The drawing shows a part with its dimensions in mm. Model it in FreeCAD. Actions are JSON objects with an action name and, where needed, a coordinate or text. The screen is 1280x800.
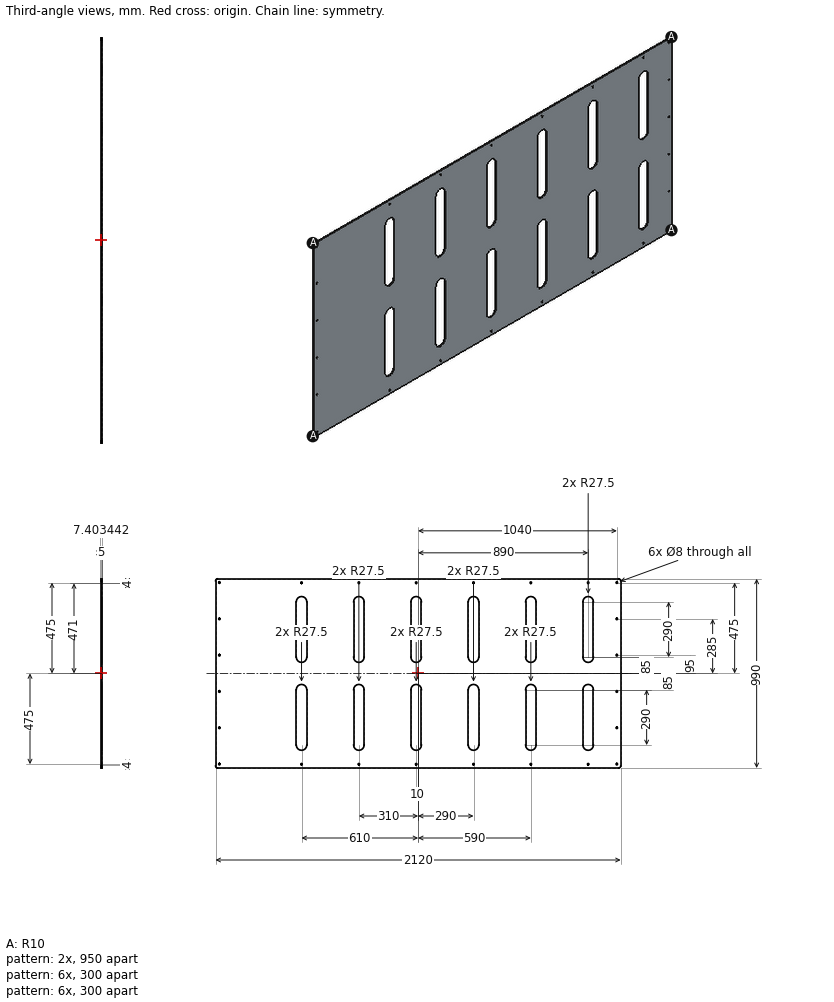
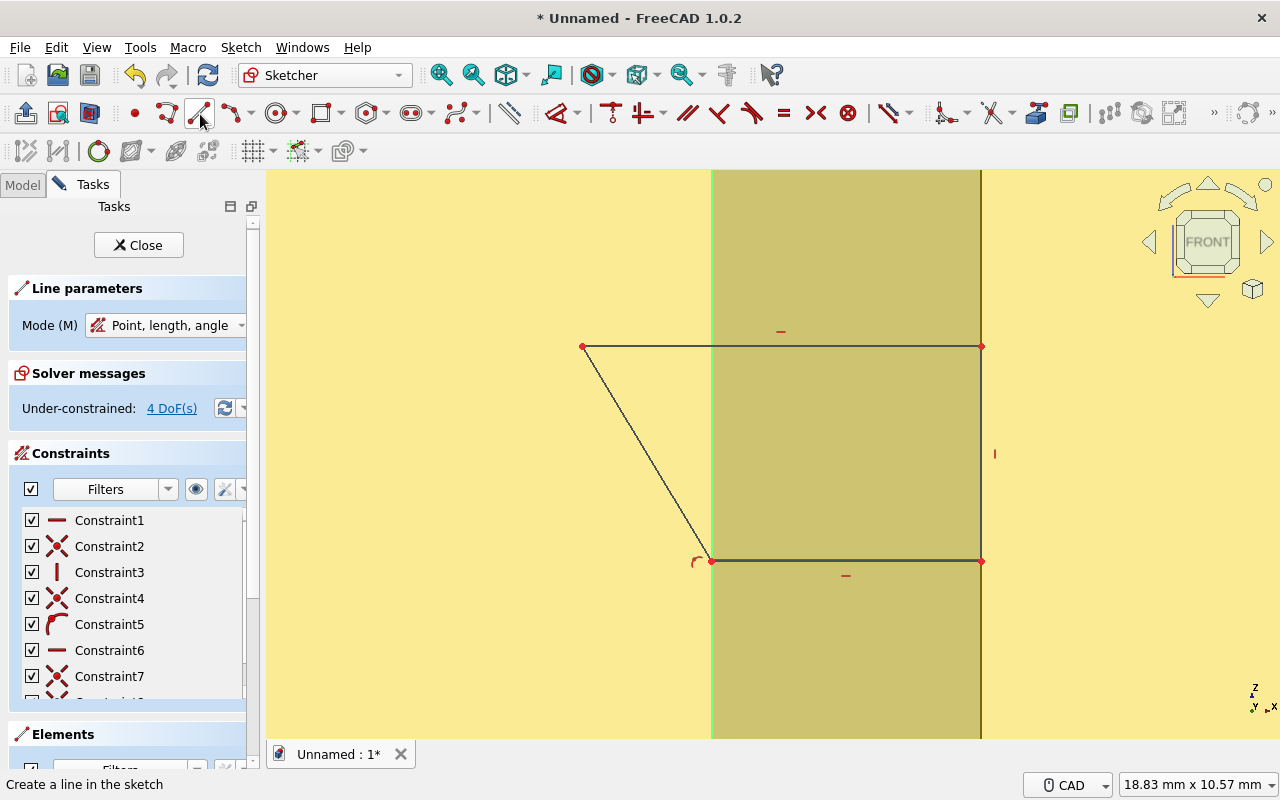
{"action": "left_click", "coordinate": [542, 345]}
{"action": "left_click", "coordinate": [423, 345]}
{"action": "key", "text": "Escape"}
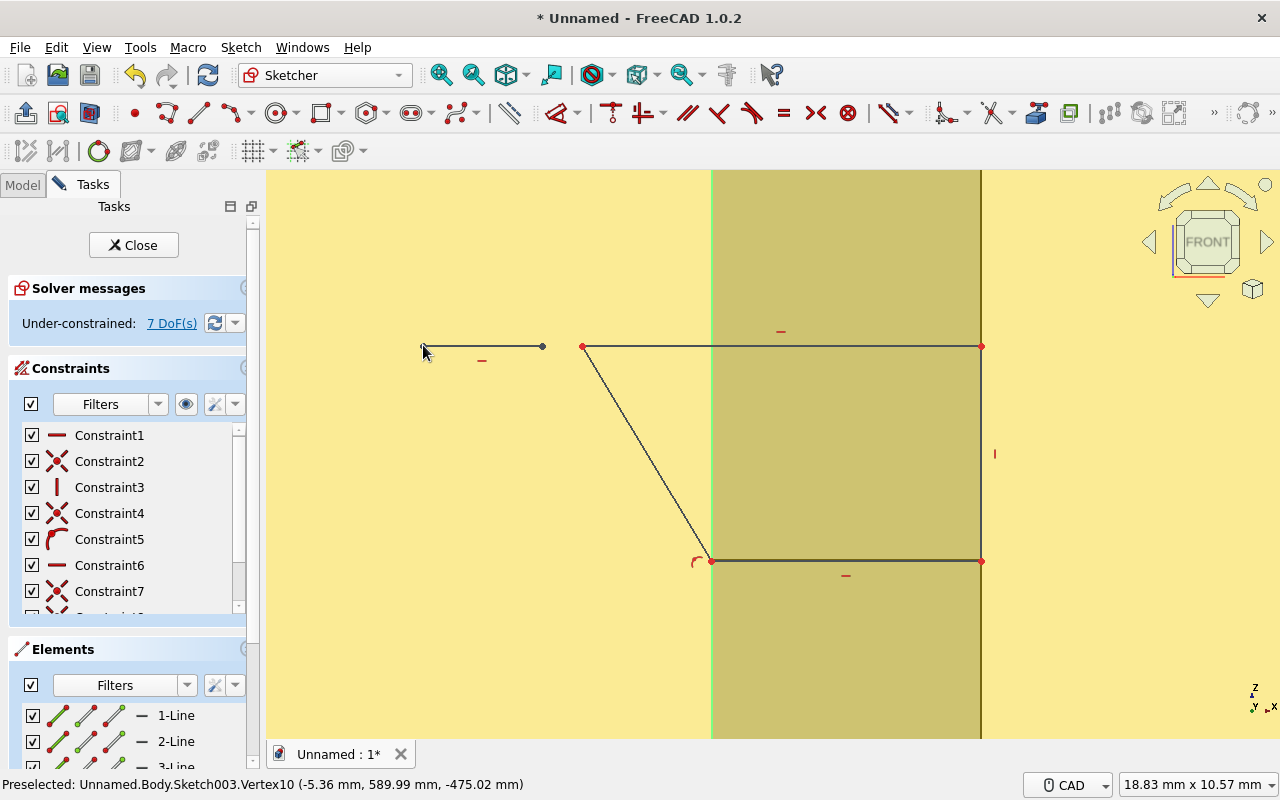
{"action": "left_click", "coordinate": [506, 346]}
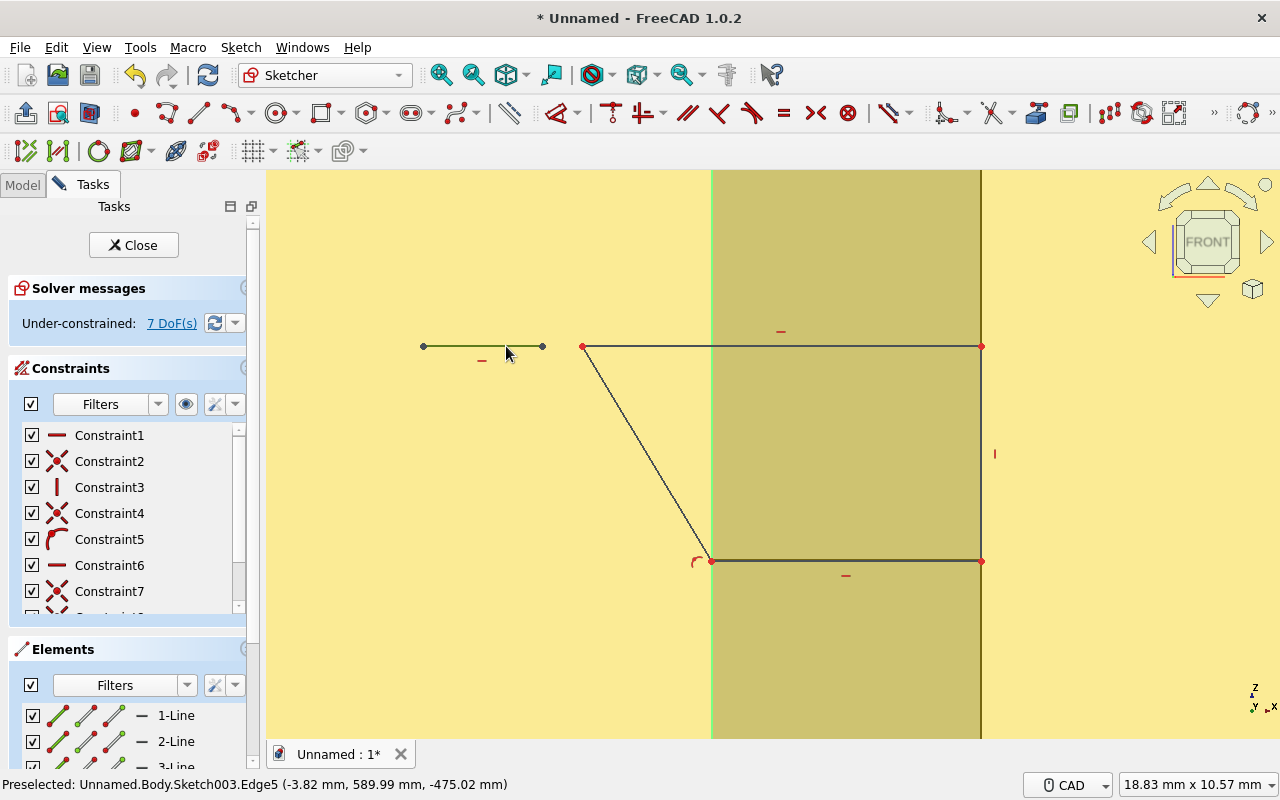
{"action": "key", "text": "g n"}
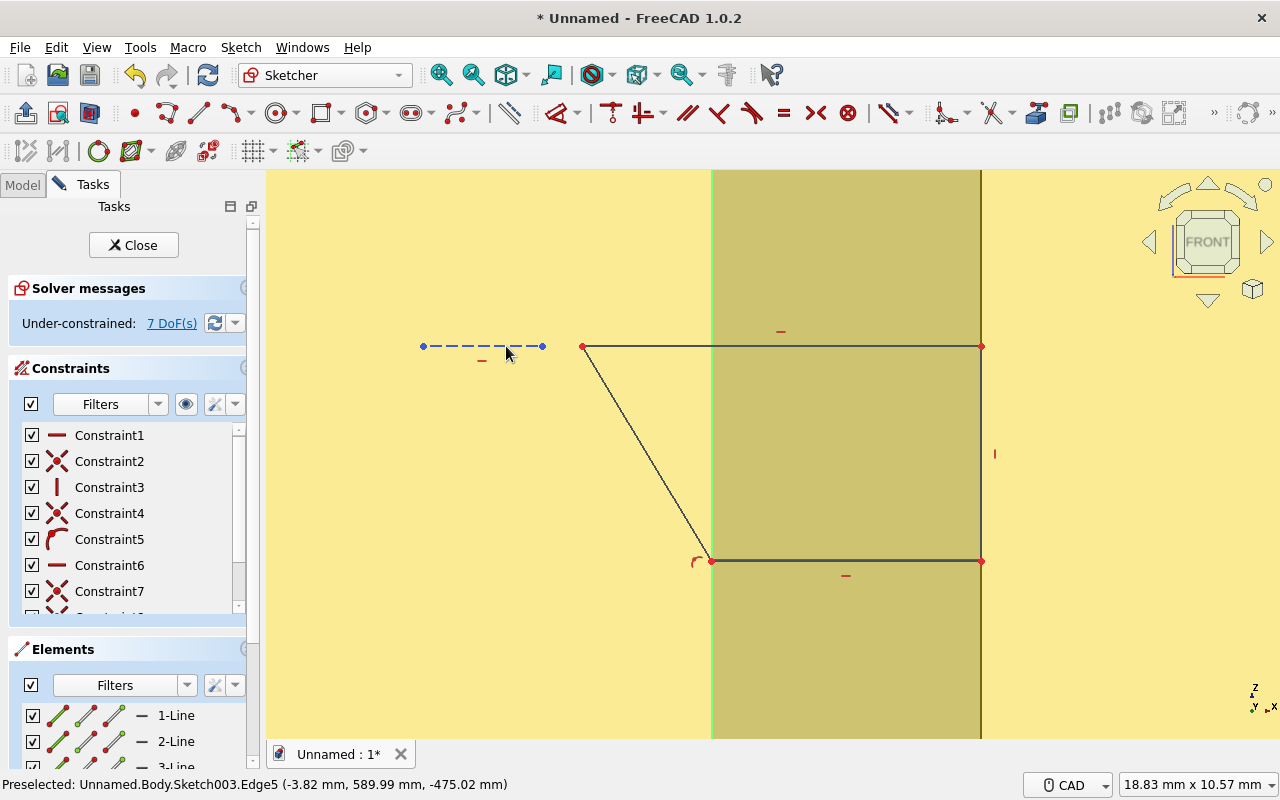
{"action": "key", "text": "d"}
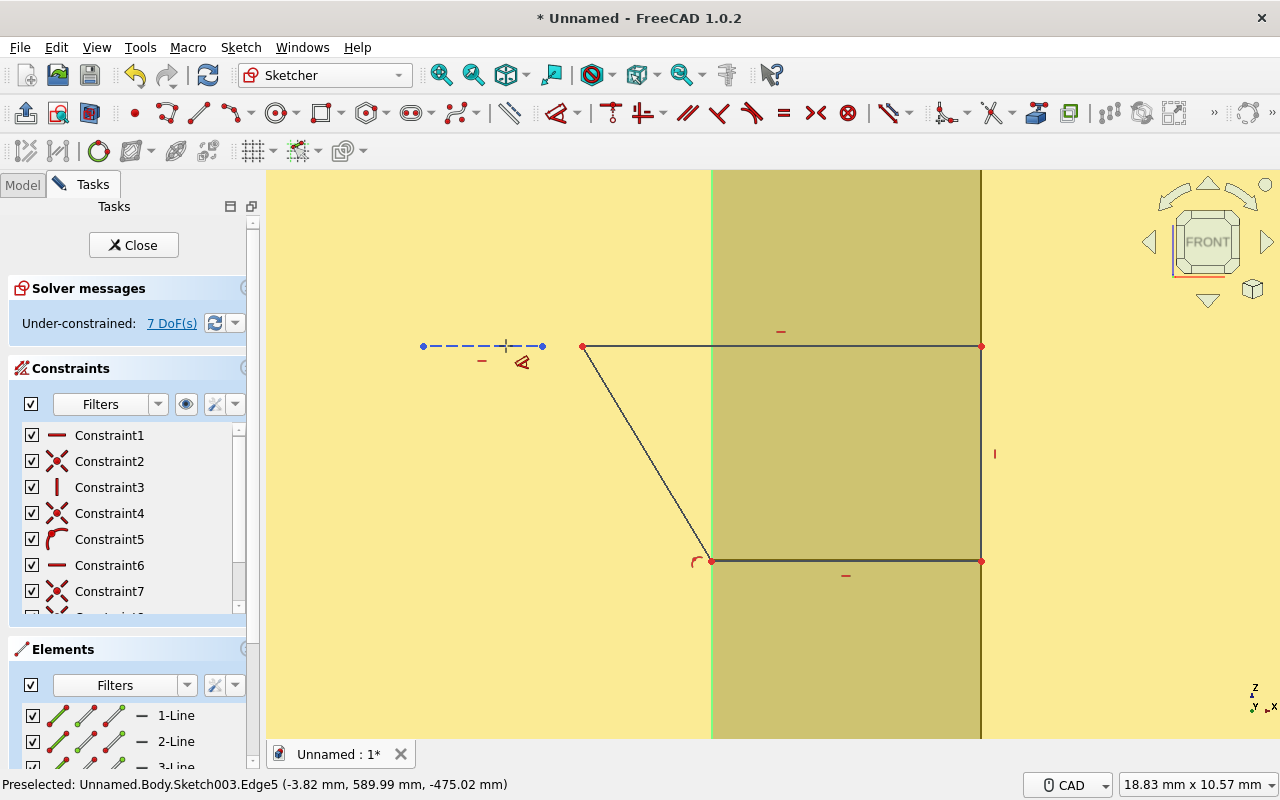
{"action": "left_click", "coordinate": [981, 411]}
{"action": "left_click", "coordinate": [1015, 454]}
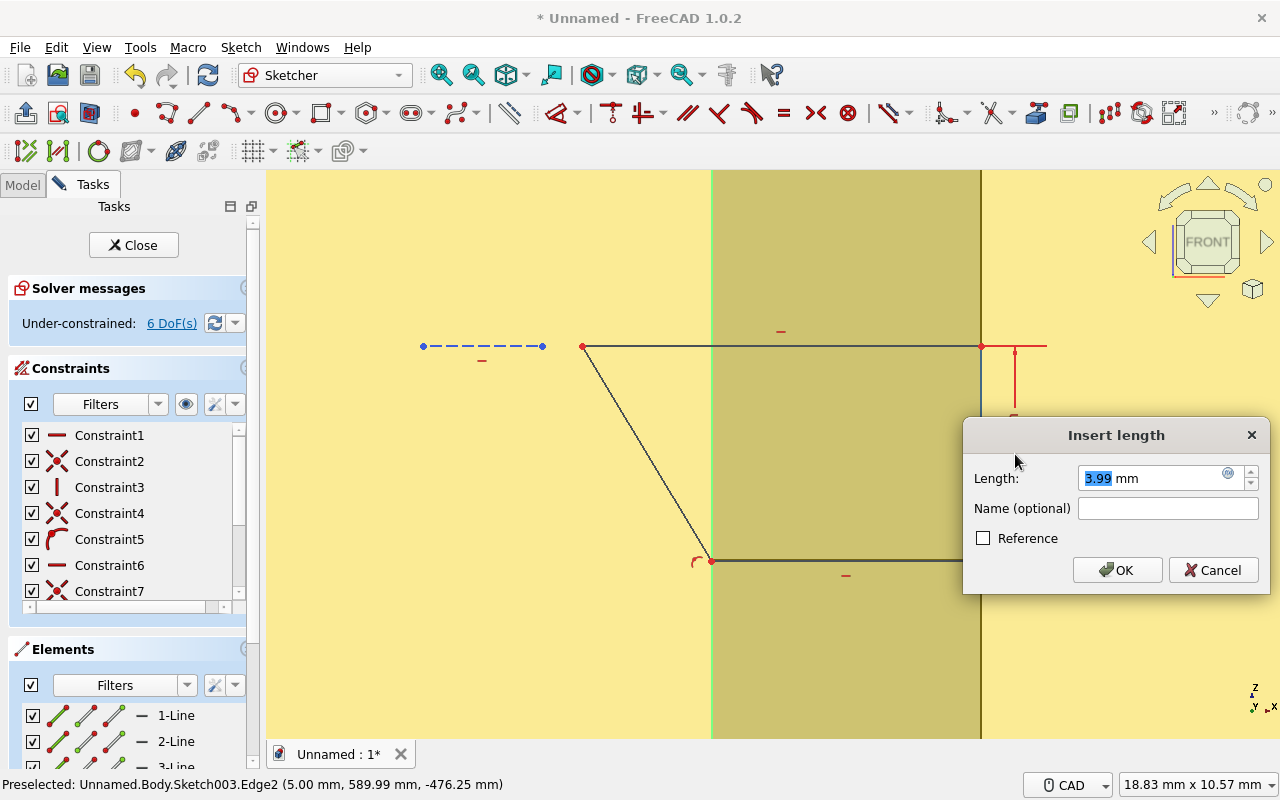
{"action": "type", "text": "4"}
{"action": "key", "text": "Return"}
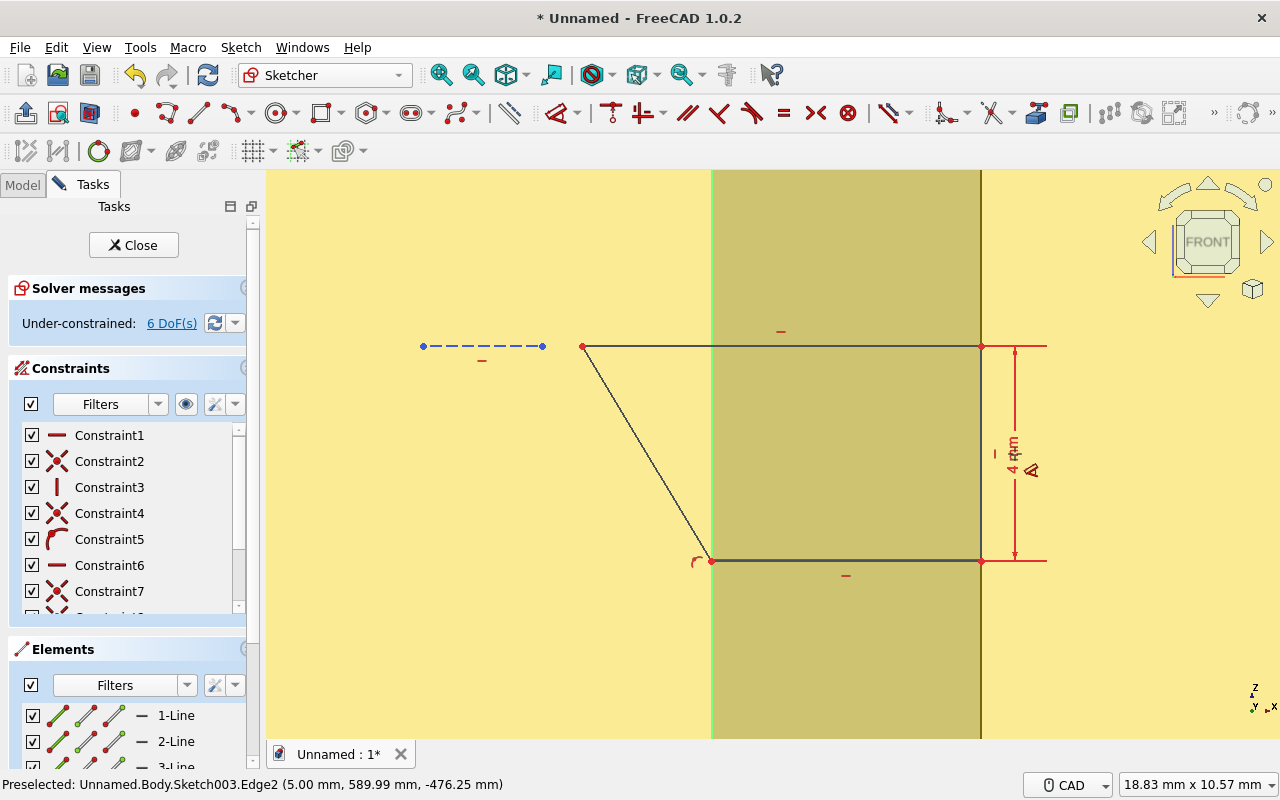
{"action": "left_click", "coordinate": [900, 561]}
{"action": "left_click", "coordinate": [846, 595]}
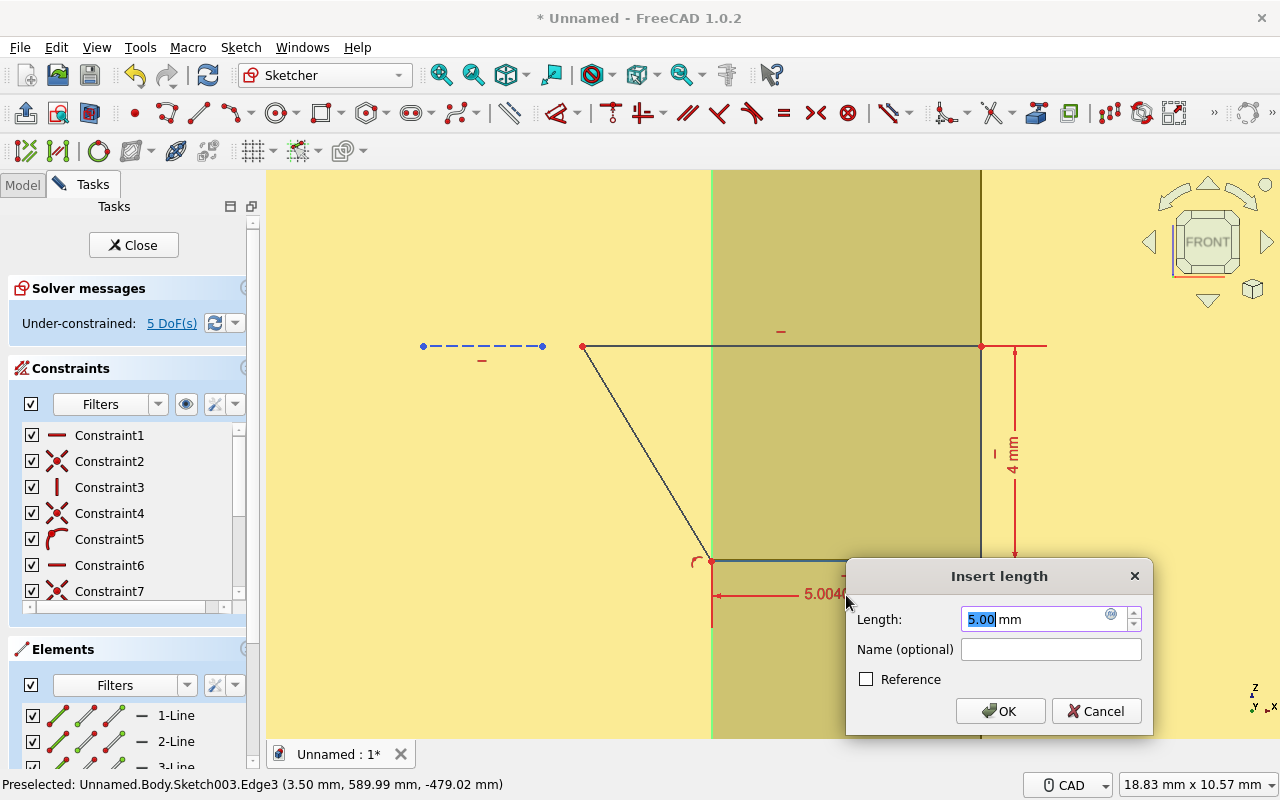
{"action": "type", "text": "5"}
{"action": "key", "text": "Return"}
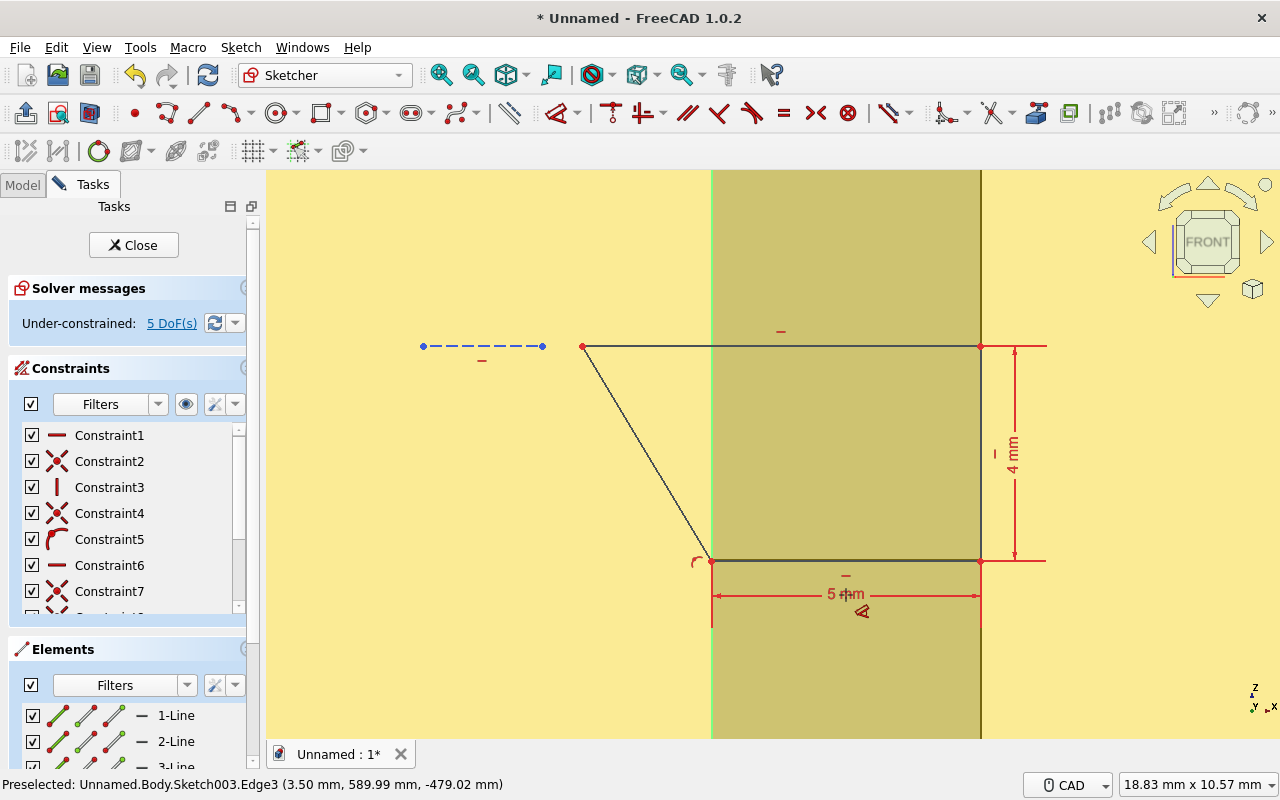
{"action": "left_click", "coordinate": [582, 346]}
{"action": "left_click", "coordinate": [548, 272]}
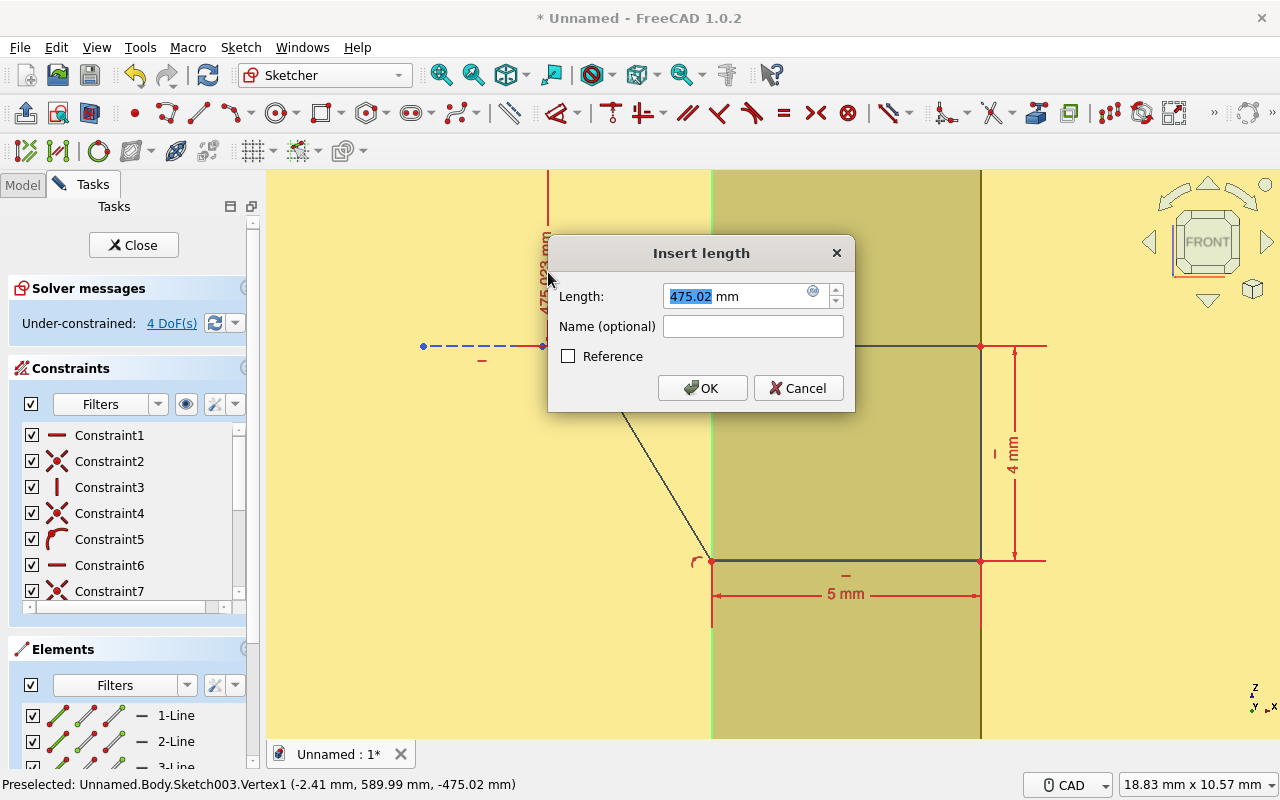
{"action": "type", "text": "475"}
{"action": "key", "text": "Return"}